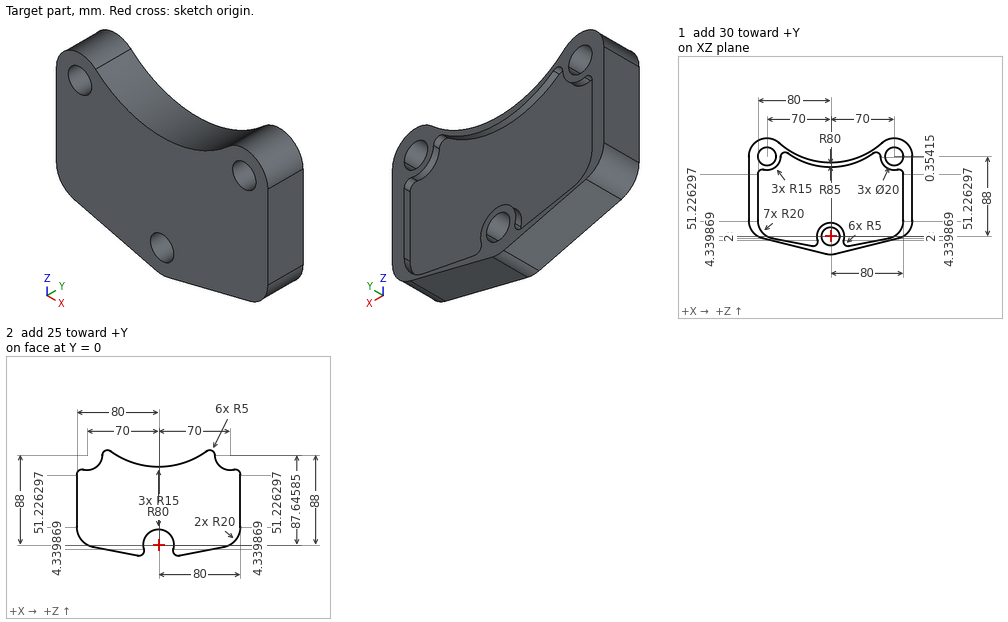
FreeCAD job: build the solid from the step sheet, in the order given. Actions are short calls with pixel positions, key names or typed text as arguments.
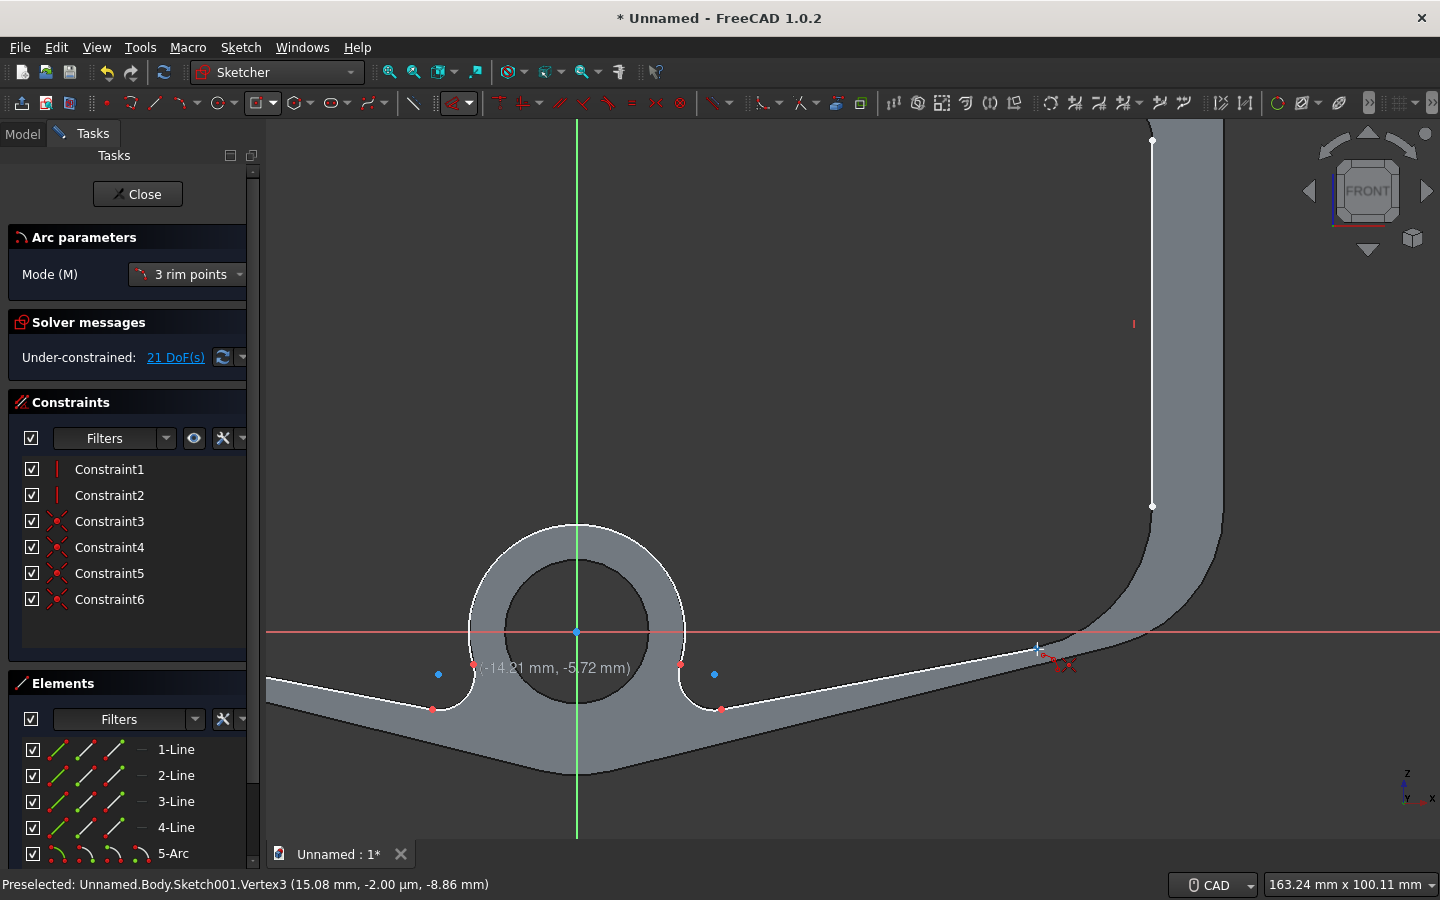
click(1036, 649)
click(1152, 507)
click(1119, 598)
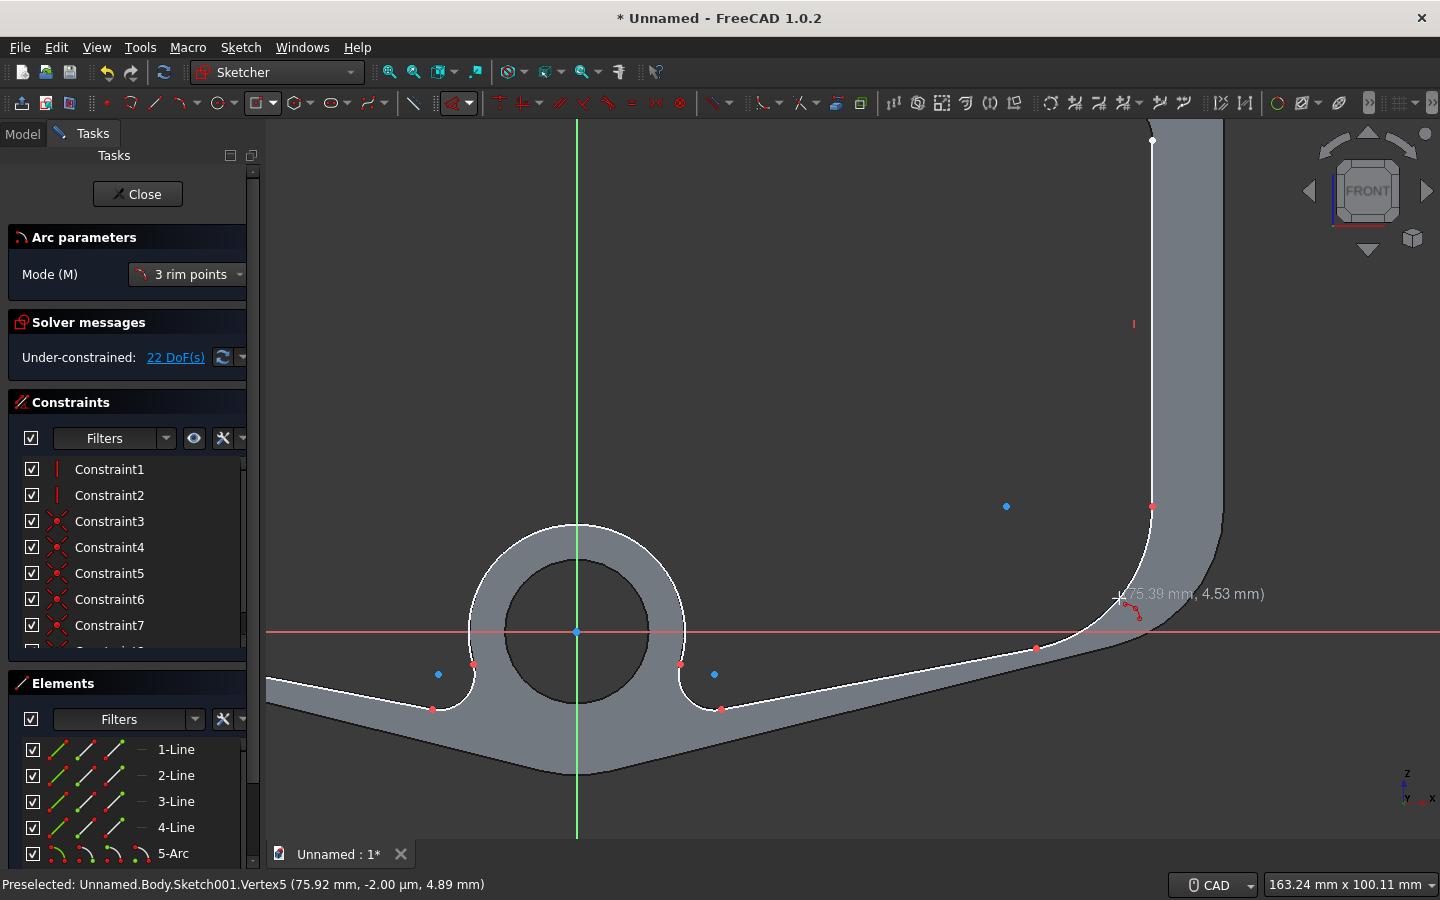
scroll(1037, 649, down, 3)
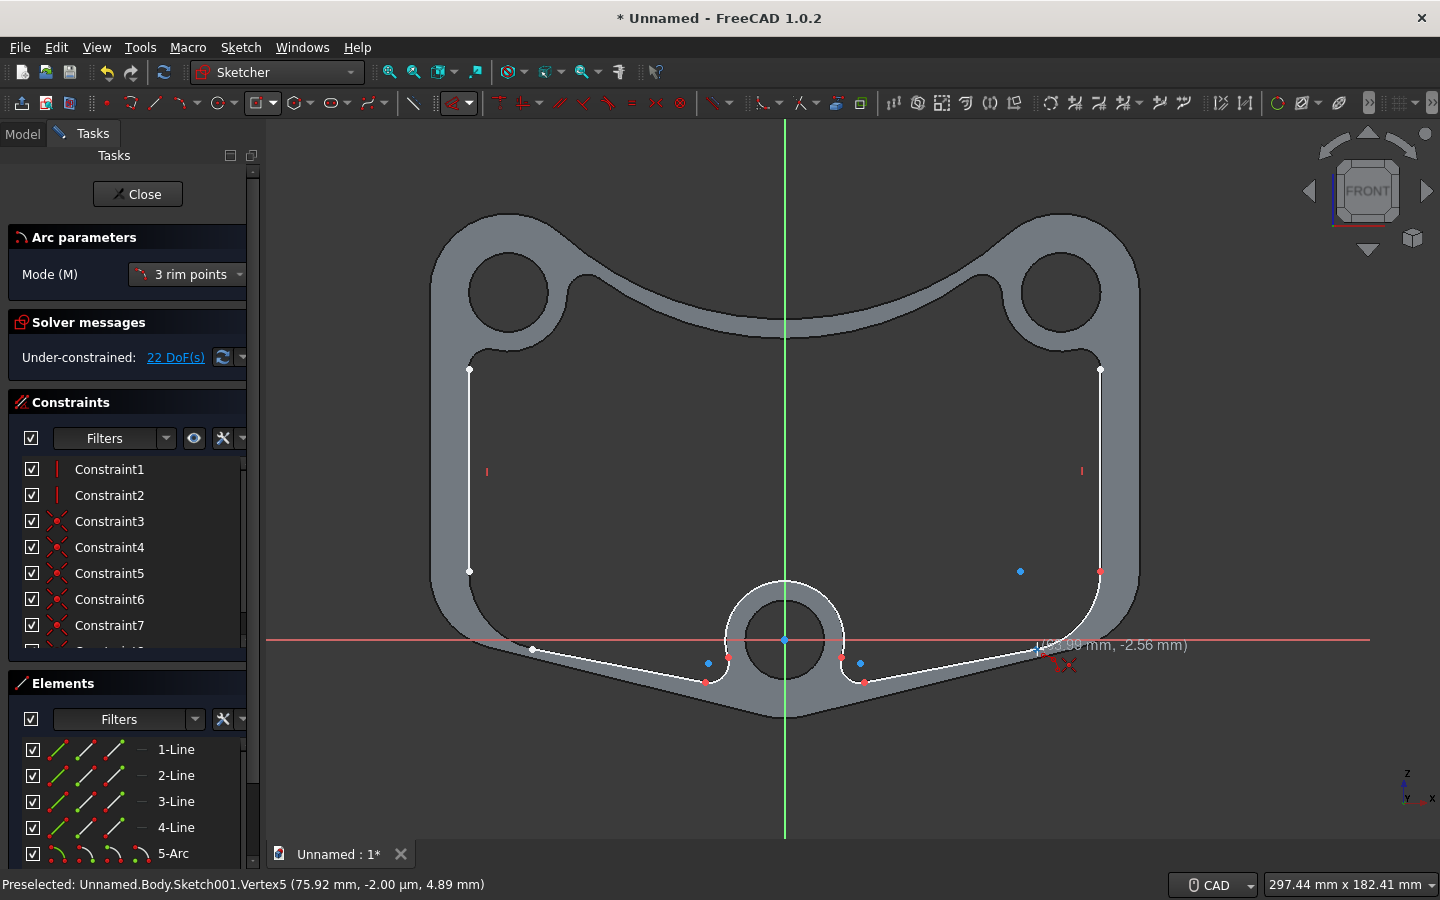
click(1100, 370)
click(1076, 350)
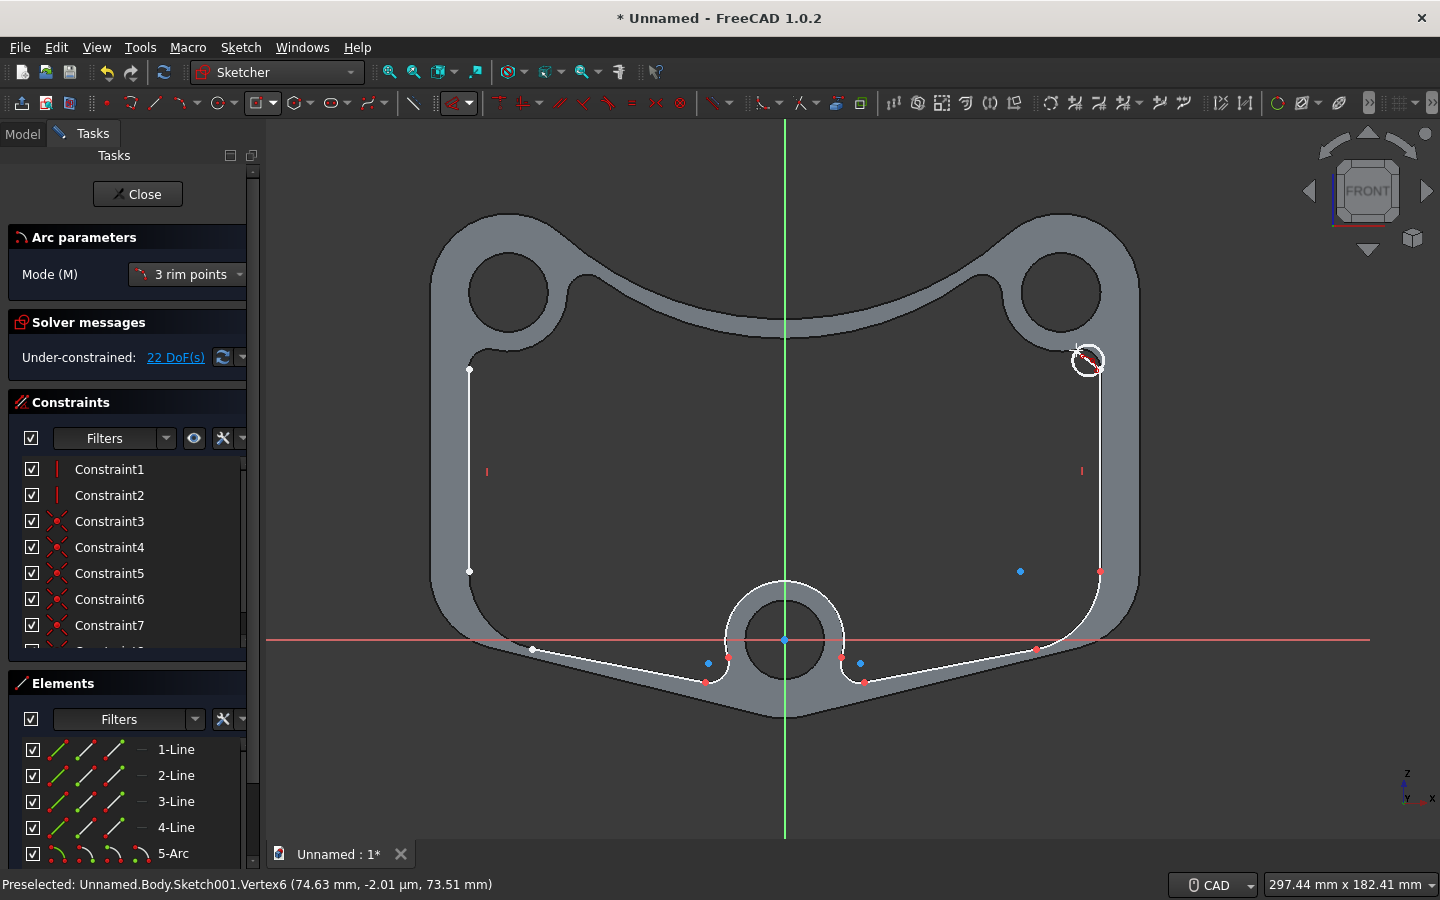
scroll(1093, 353, up, 4)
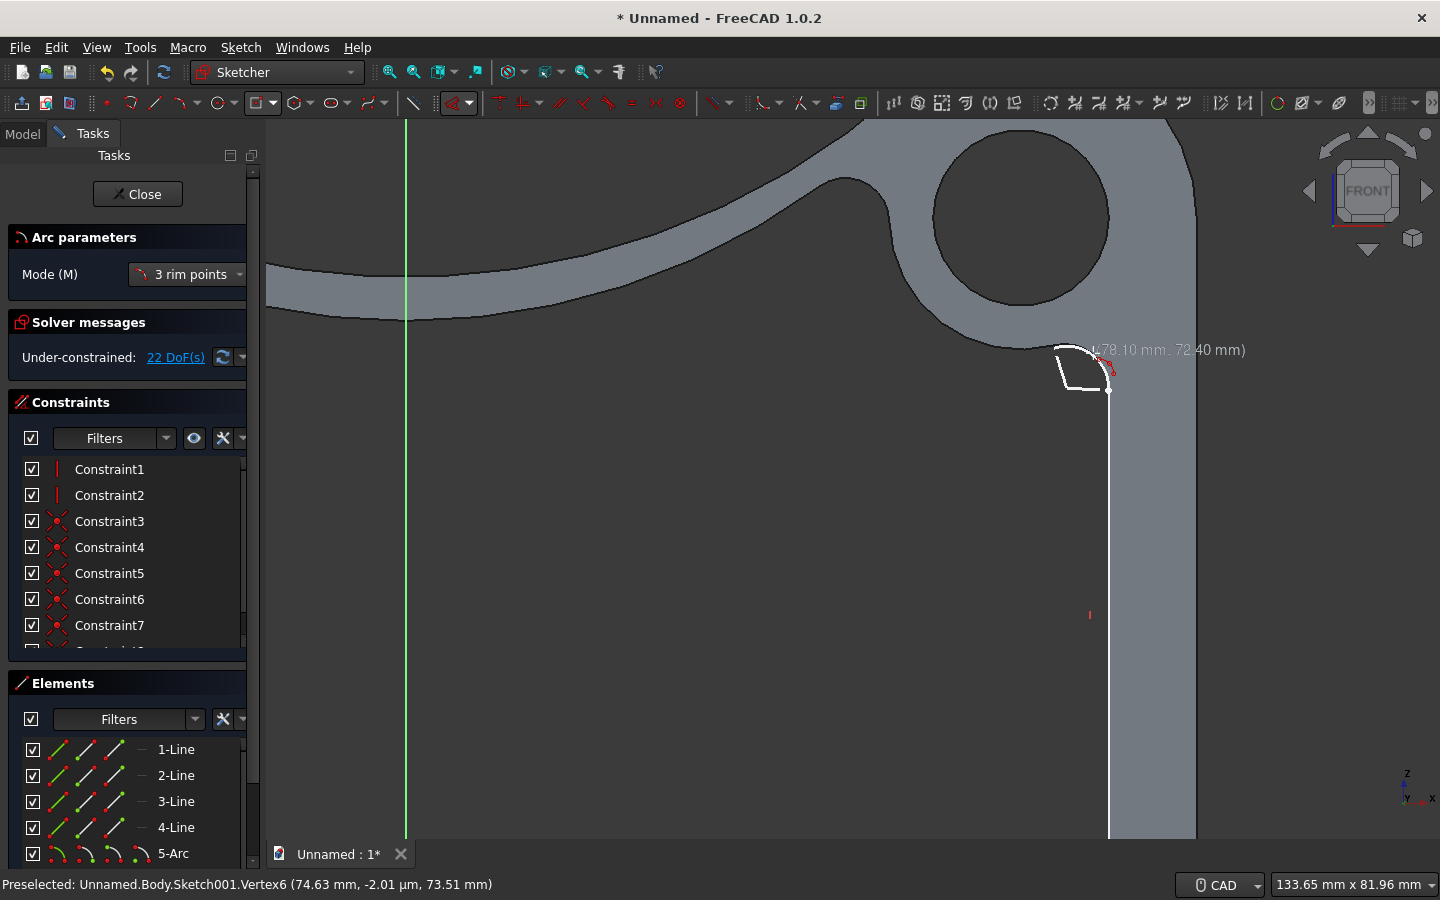
click(1092, 353)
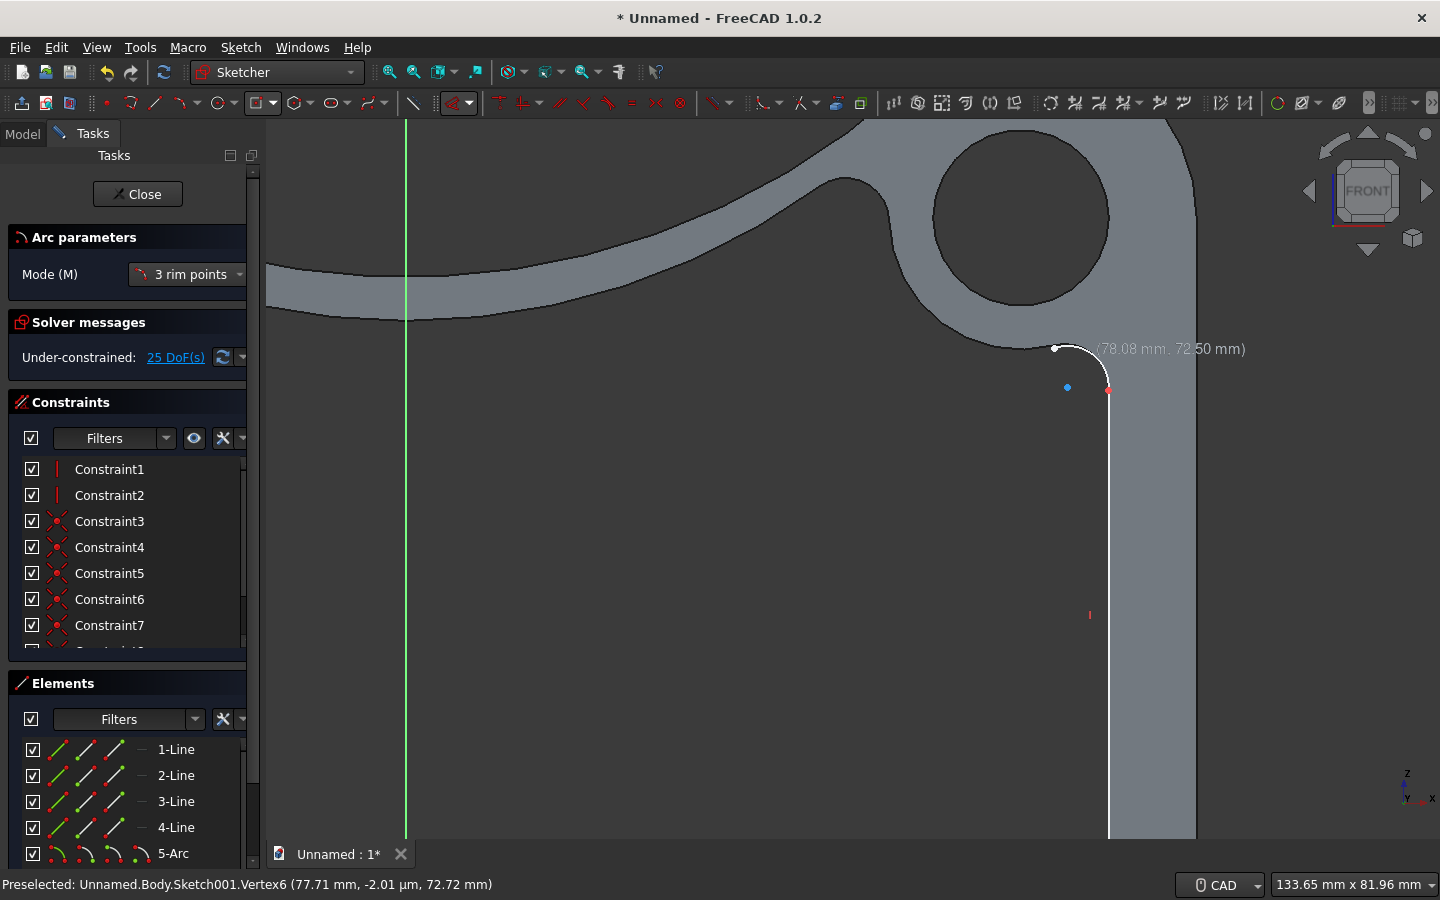
click(1054, 348)
click(889, 221)
click(942, 323)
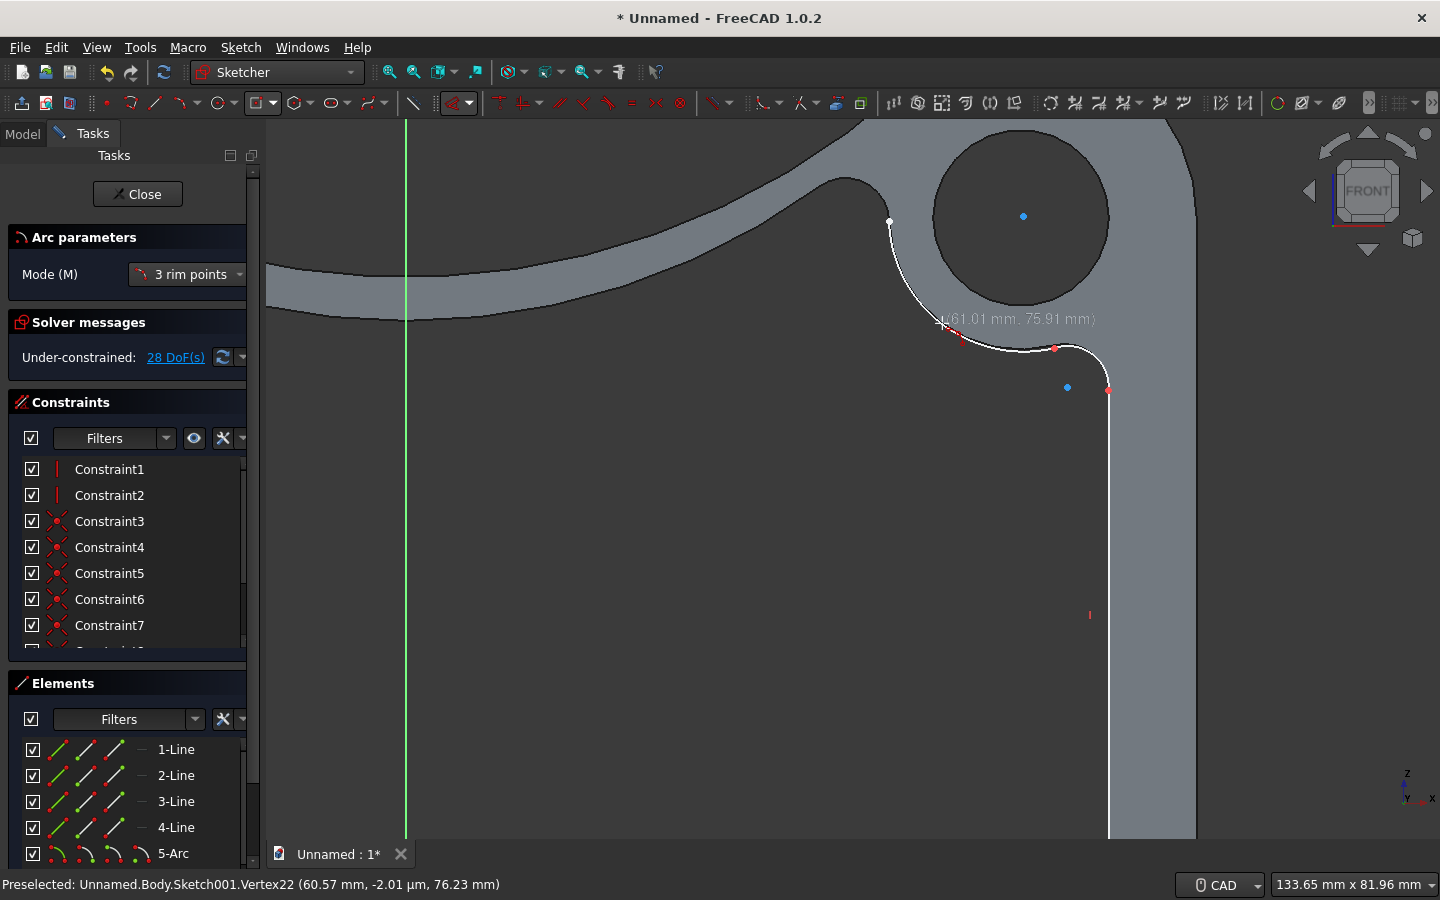
click(889, 222)
click(820, 186)
click(865, 183)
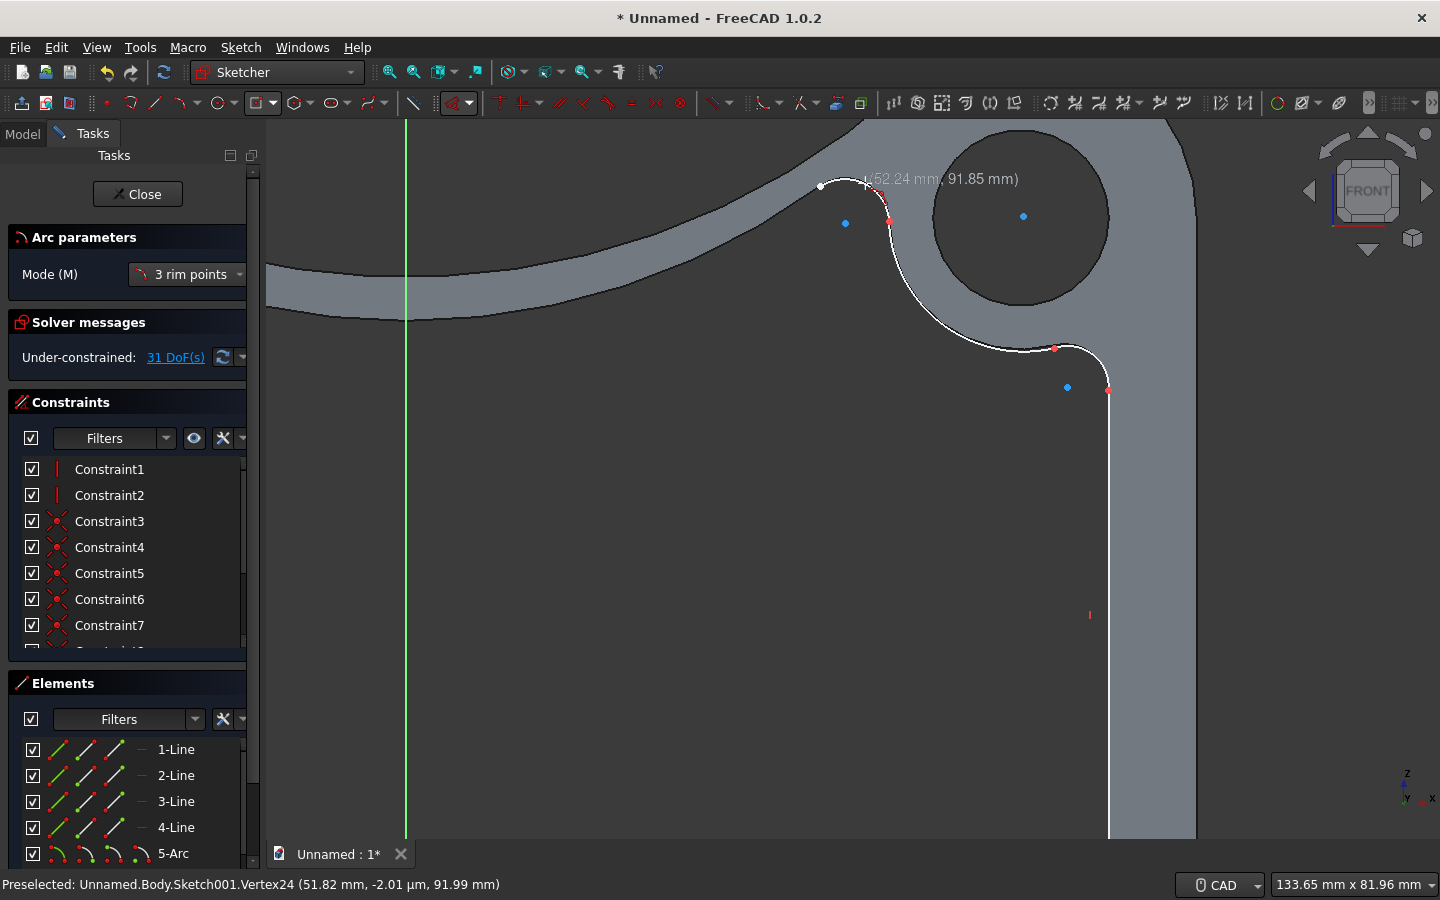
click(820, 187)